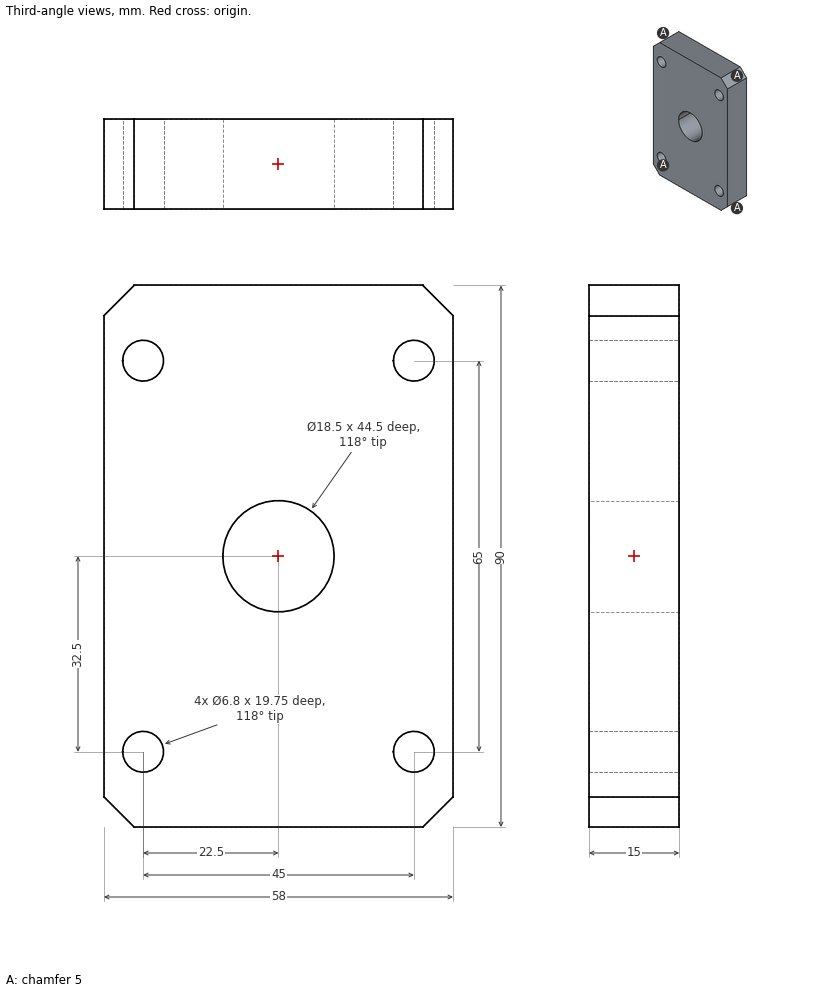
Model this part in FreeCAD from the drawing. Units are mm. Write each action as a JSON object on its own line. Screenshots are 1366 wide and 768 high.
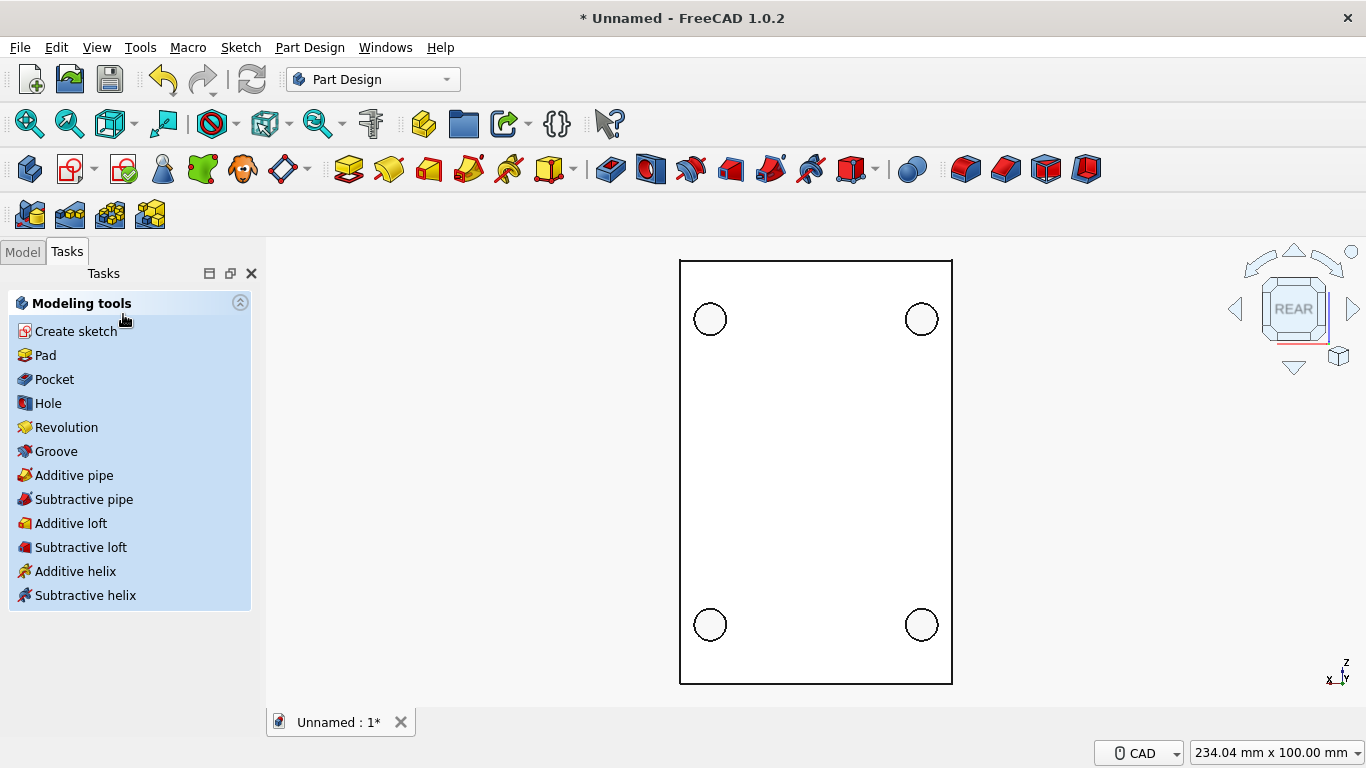
{"action": "left_click", "coordinate": [652, 170]}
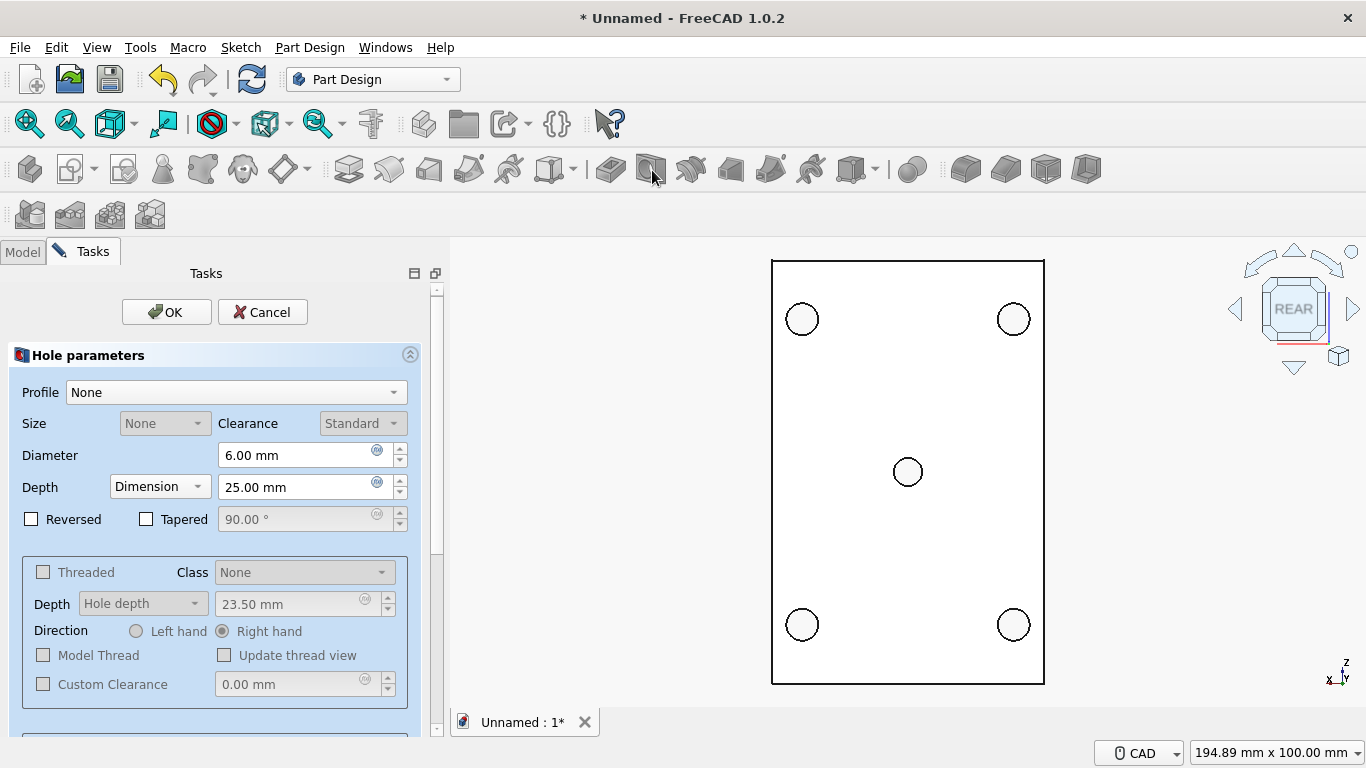
{"action": "triple_click", "coordinate": [305, 455]}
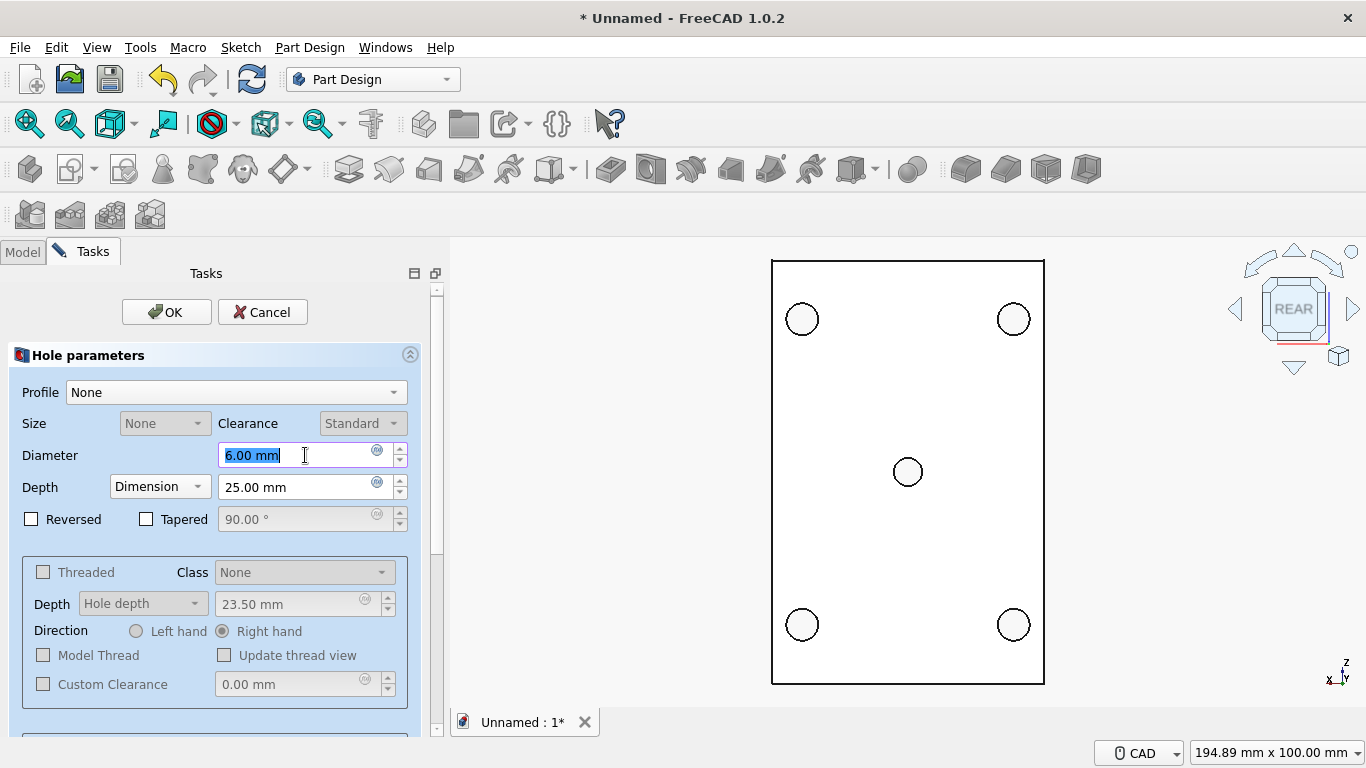
{"action": "type", "text": "18.5"}
{"action": "key", "text": "Tab"}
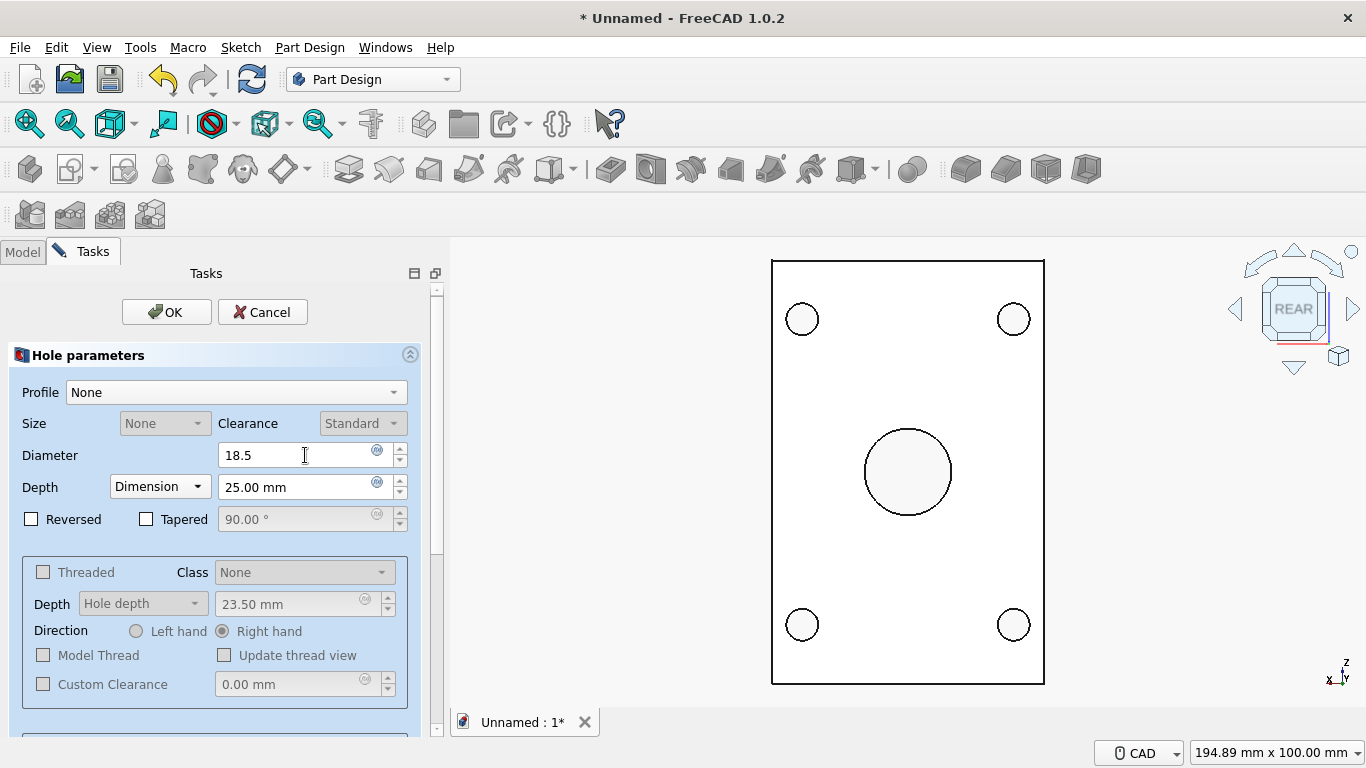
{"action": "triple_click", "coordinate": [305, 487]}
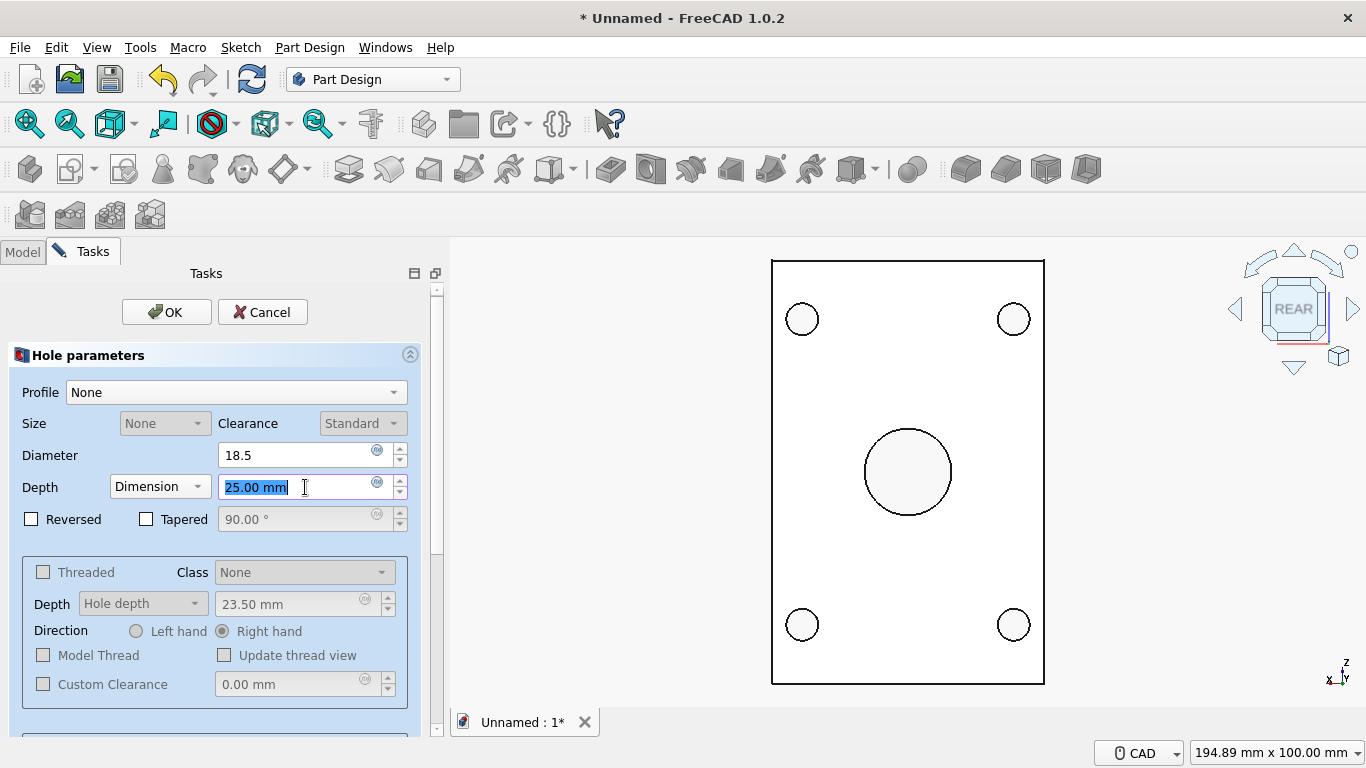
{"action": "type", "text": "44.5"}
{"action": "key", "text": "Tab"}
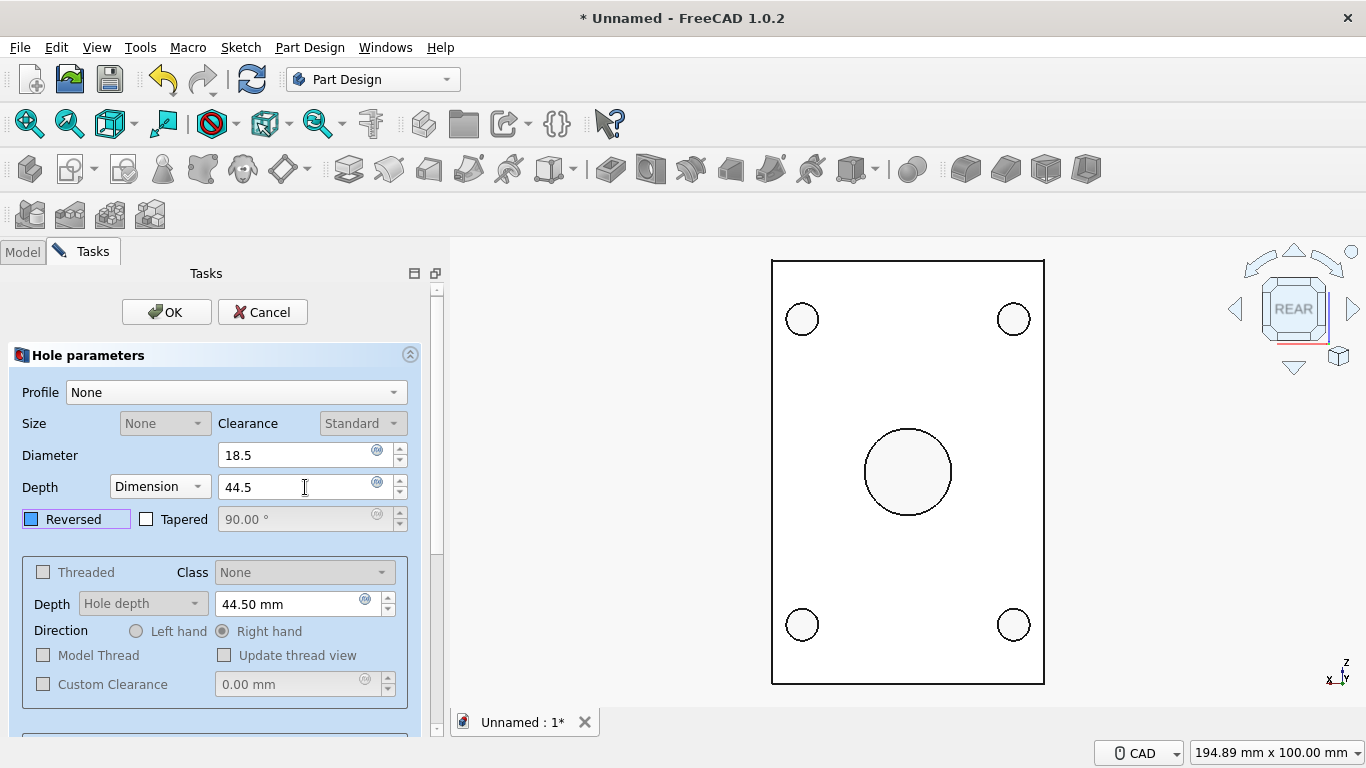
{"action": "left_click", "coordinate": [167, 312]}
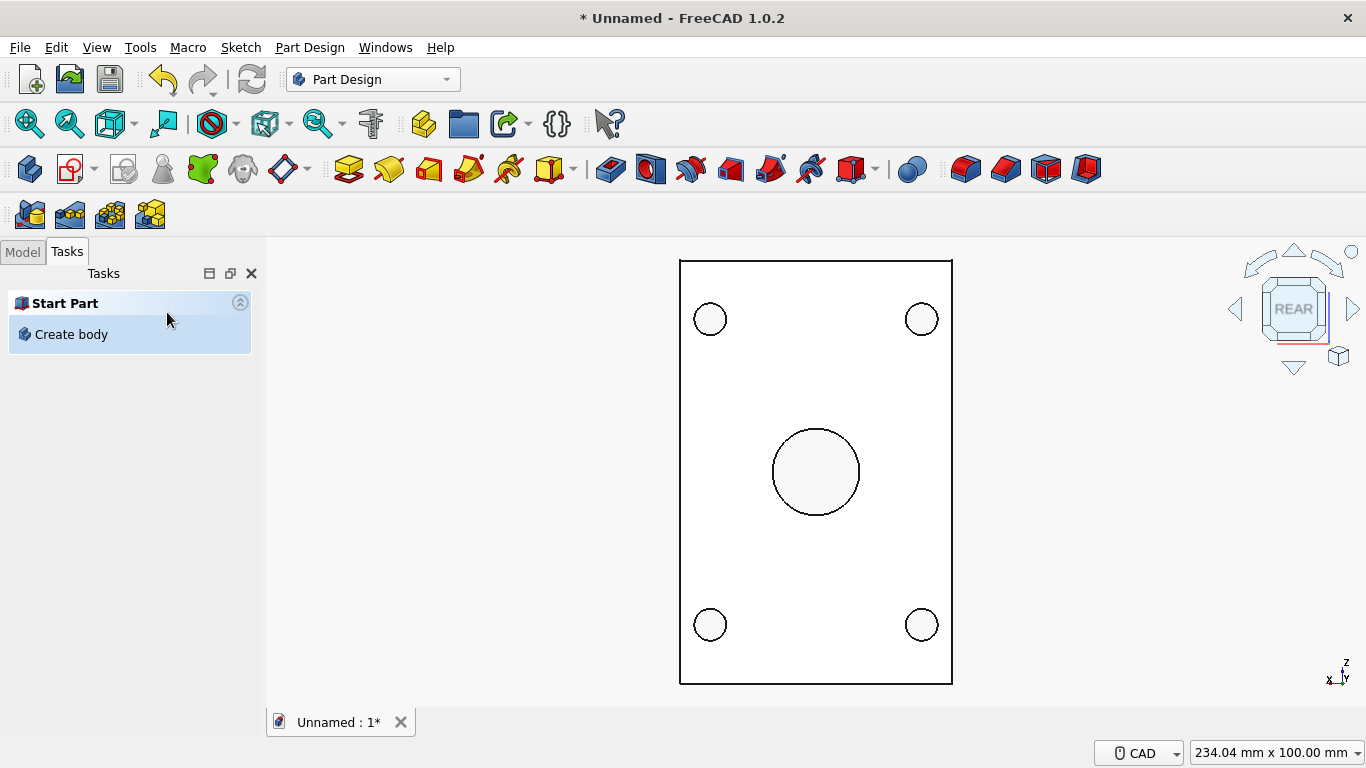
{"action": "key", "text": "0"}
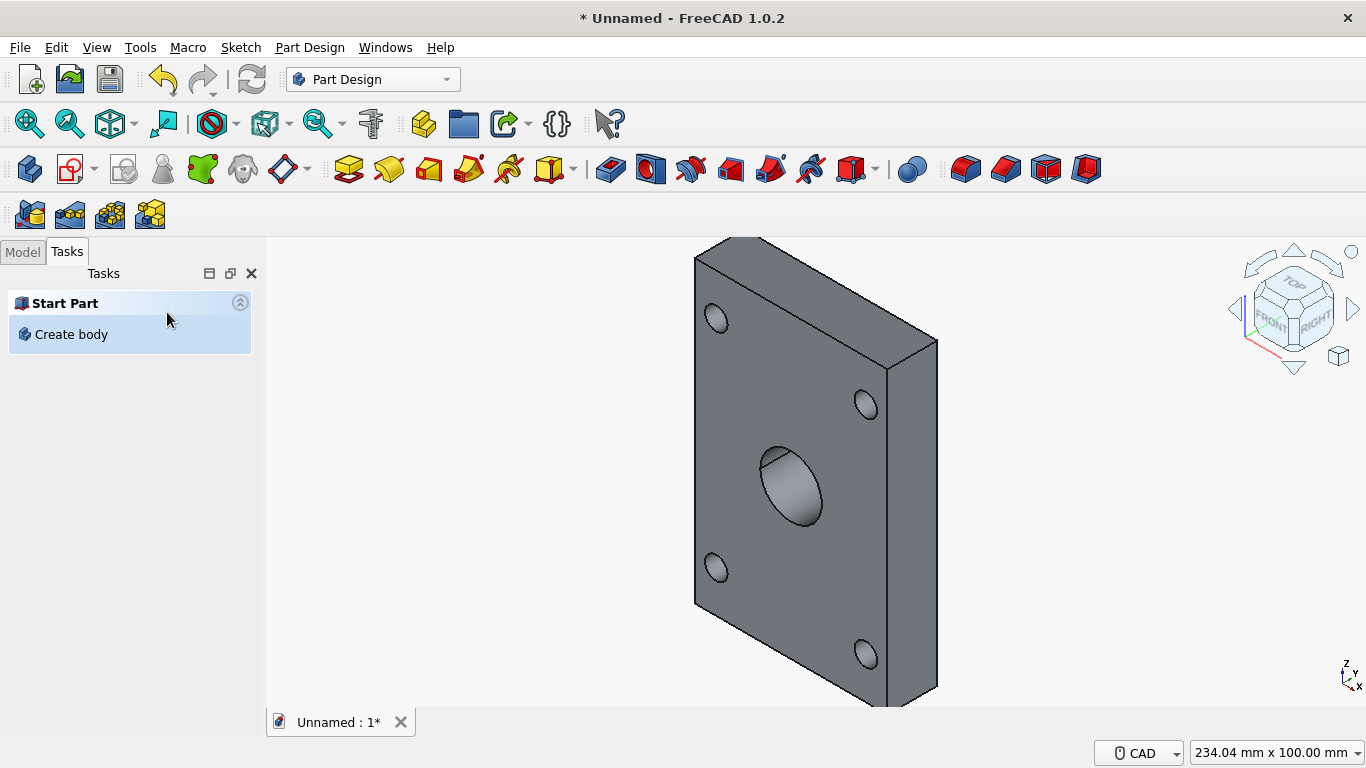
{"action": "key", "text": "v f"}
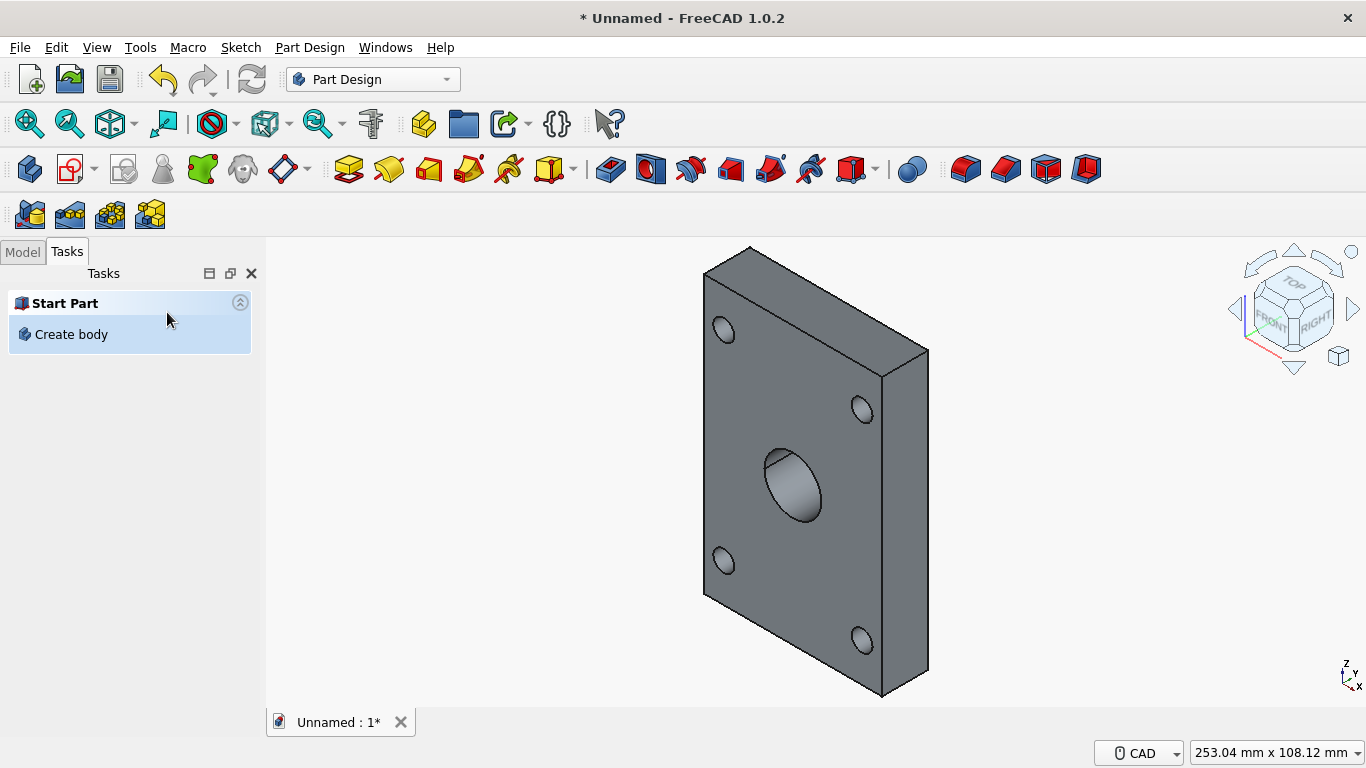
{"action": "left_click", "coordinate": [905, 363]}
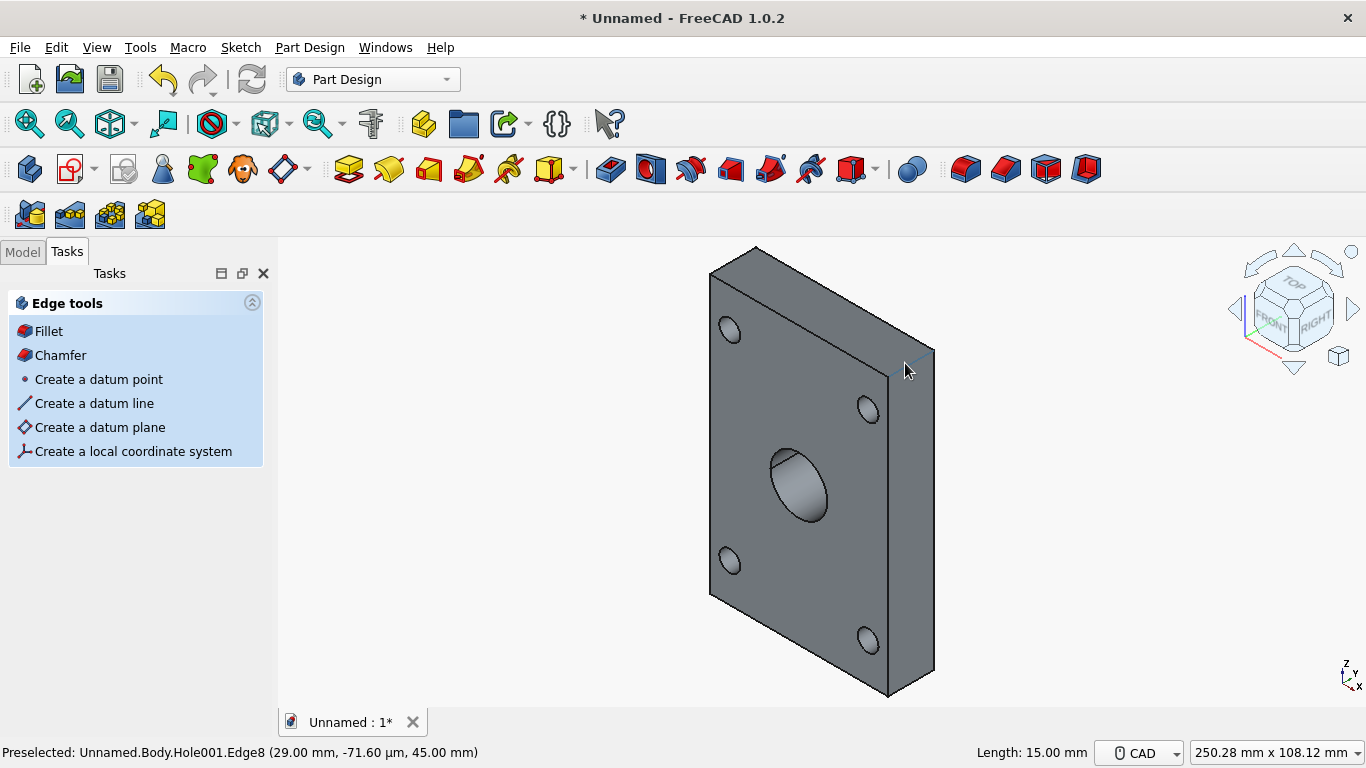
{"action": "key", "text": "2"}